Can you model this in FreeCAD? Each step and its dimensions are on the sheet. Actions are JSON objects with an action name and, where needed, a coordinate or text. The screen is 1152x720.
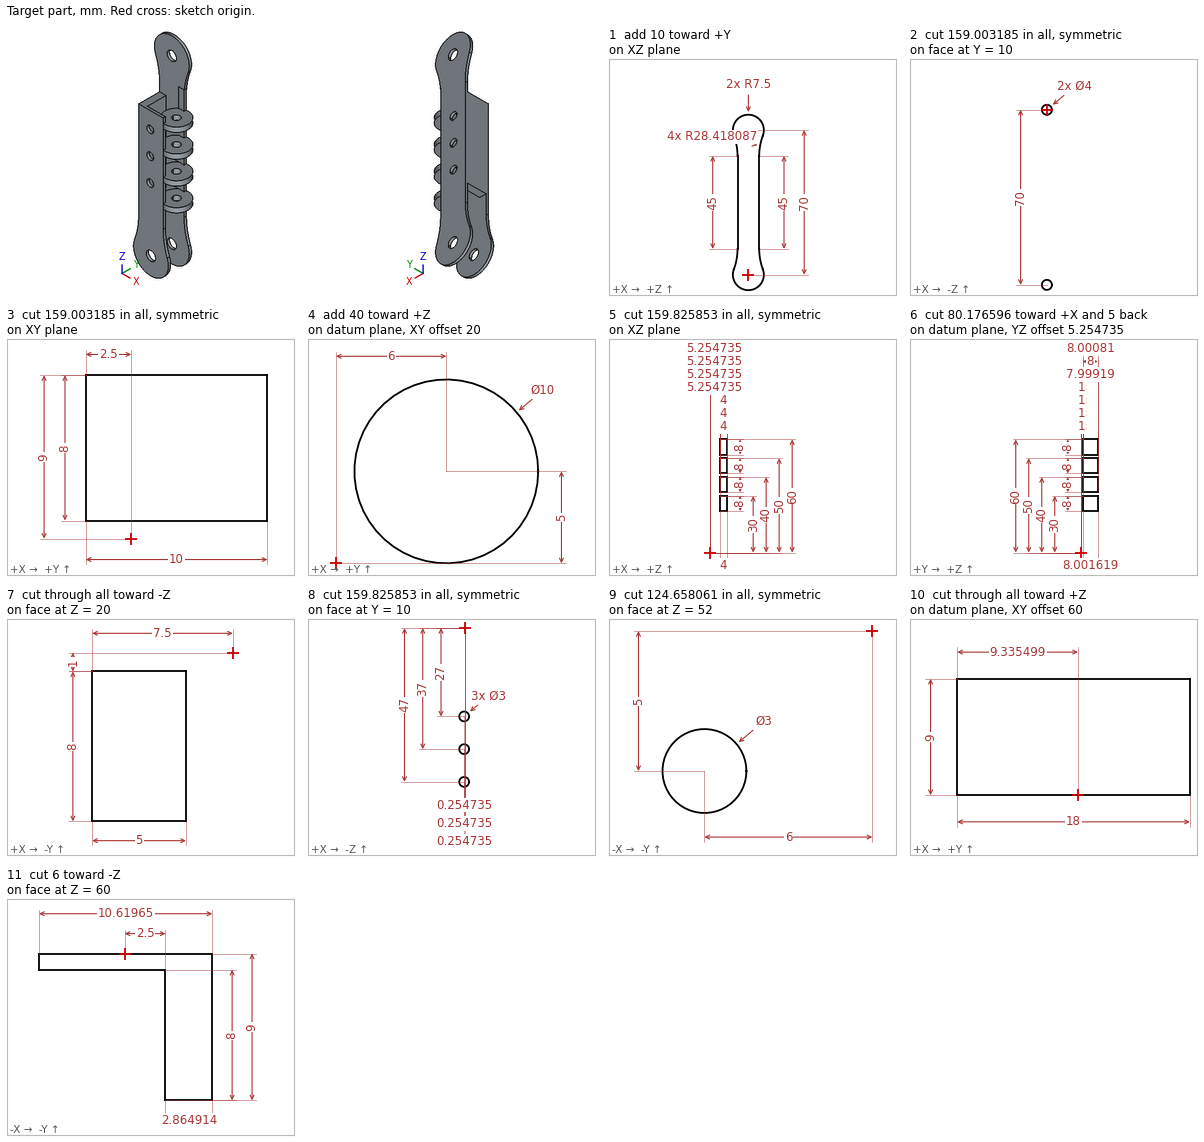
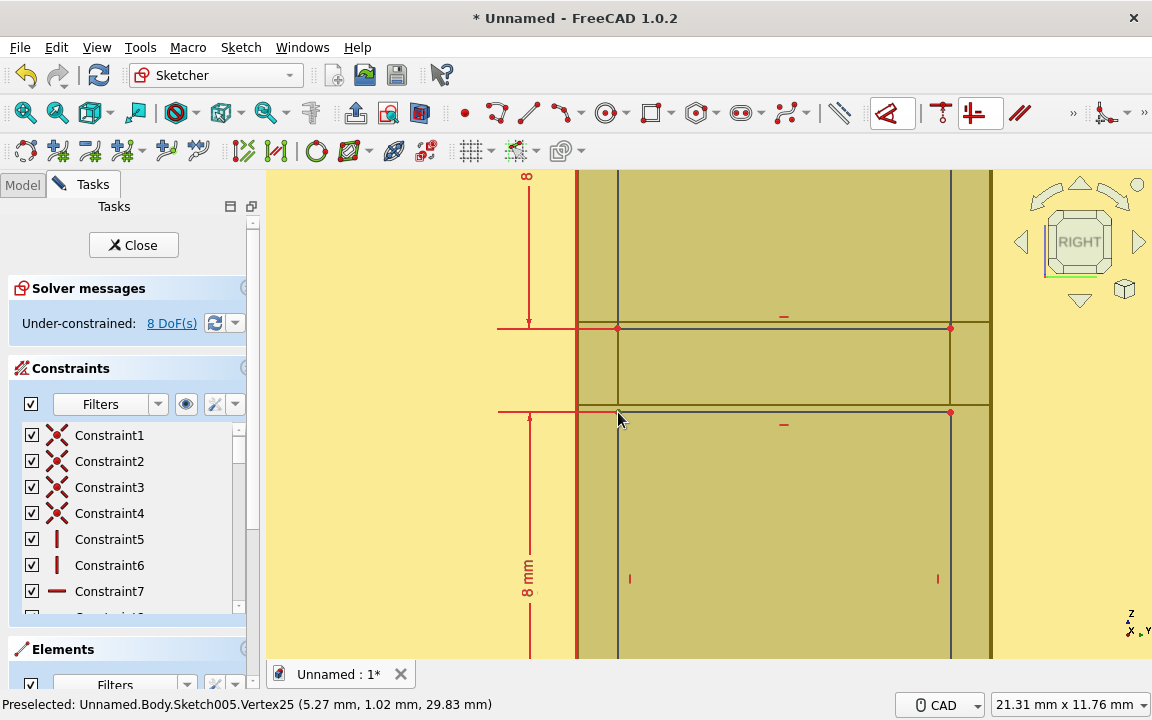
{"action": "left_click", "coordinate": [910, 114]}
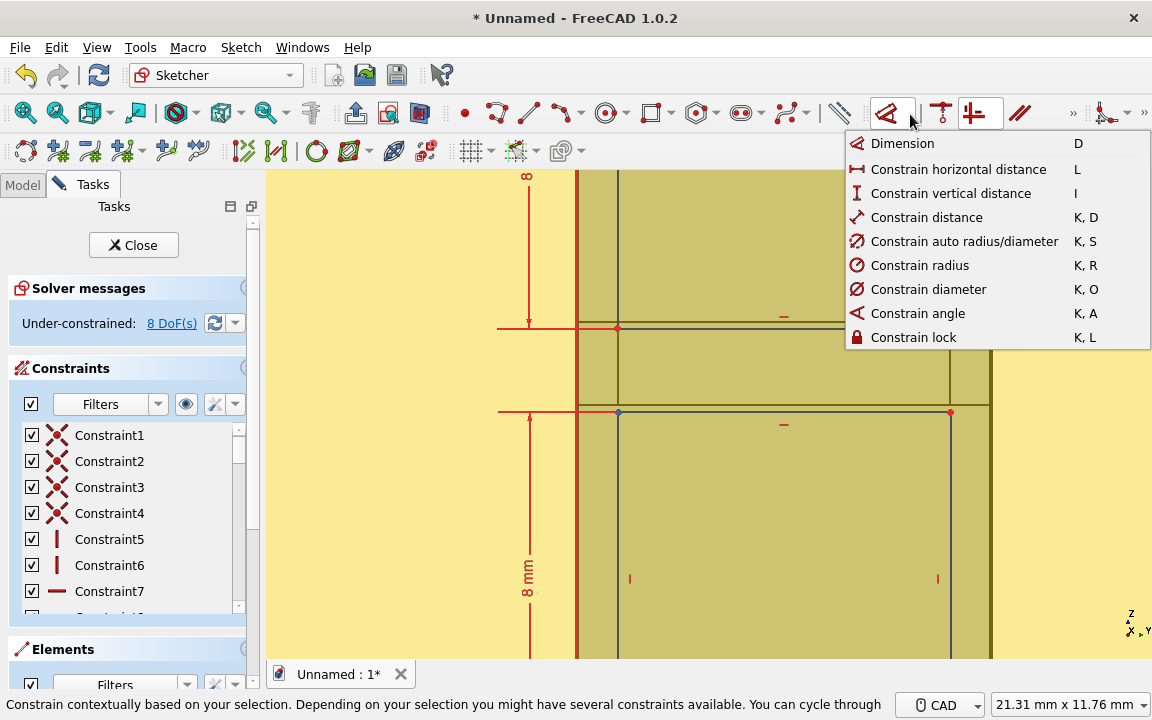
{"action": "left_click", "coordinate": [998, 169]}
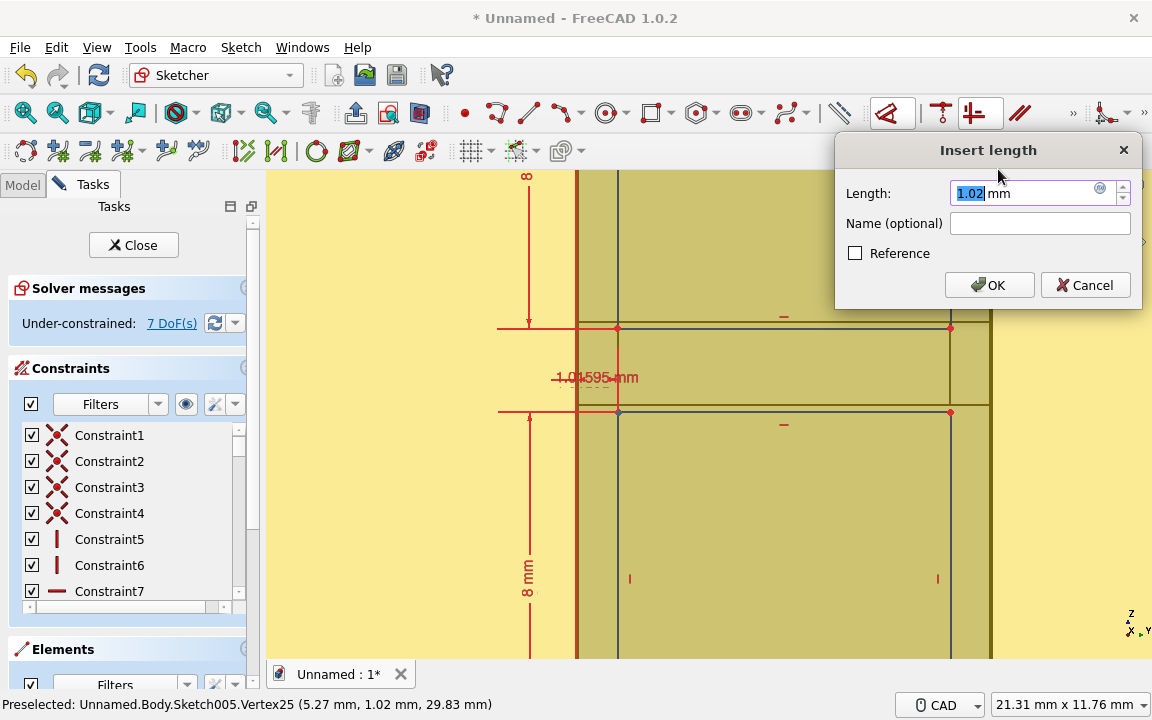
{"action": "type", "text": "1"}
{"action": "key", "text": "Return"}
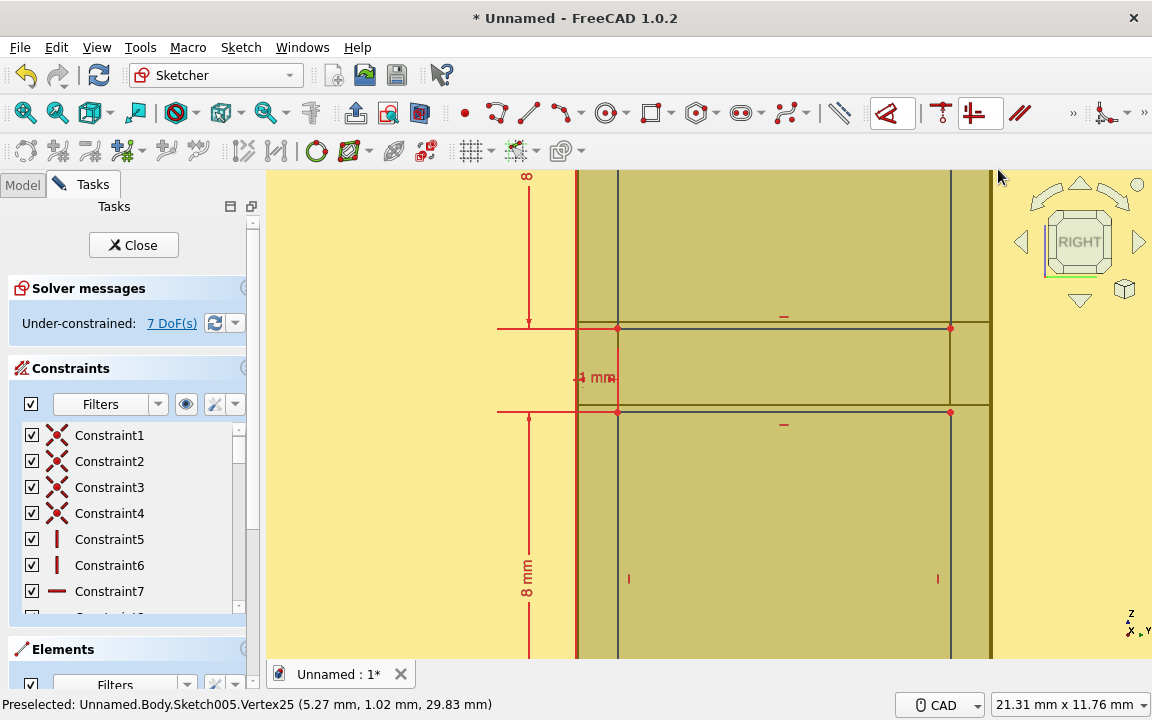
{"action": "scroll", "coordinate": [621, 416], "scroll_direction": "down", "scroll_amount": 10}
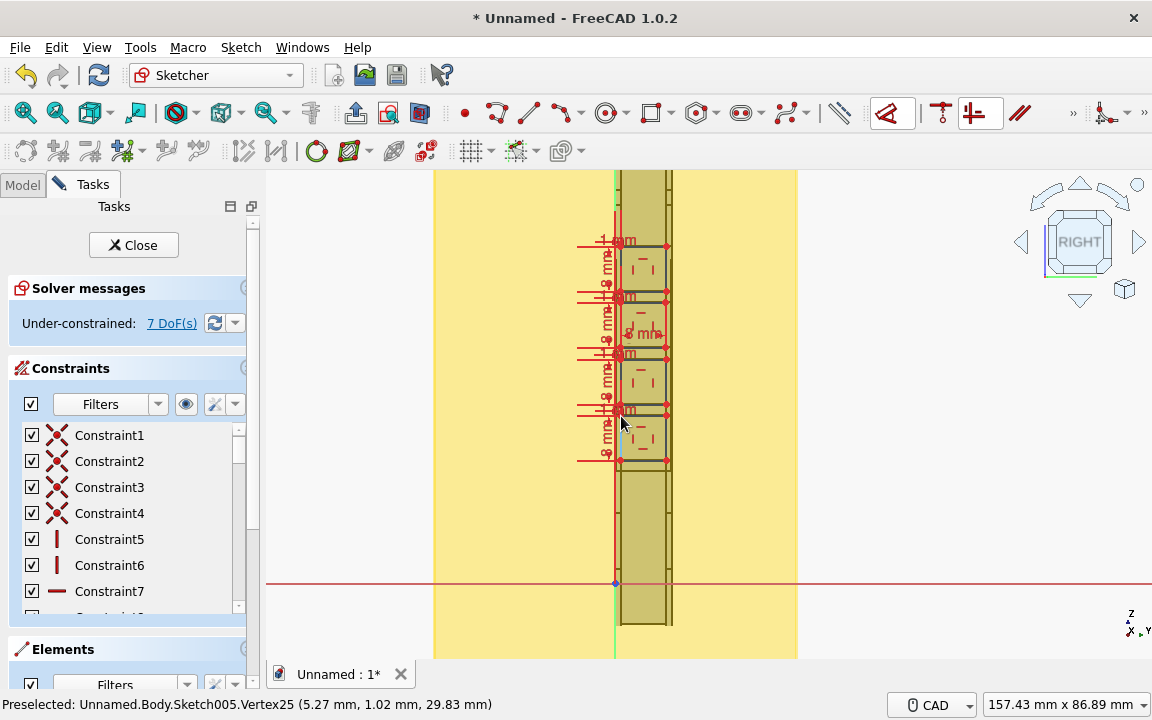
{"action": "left_click", "coordinate": [621, 247]}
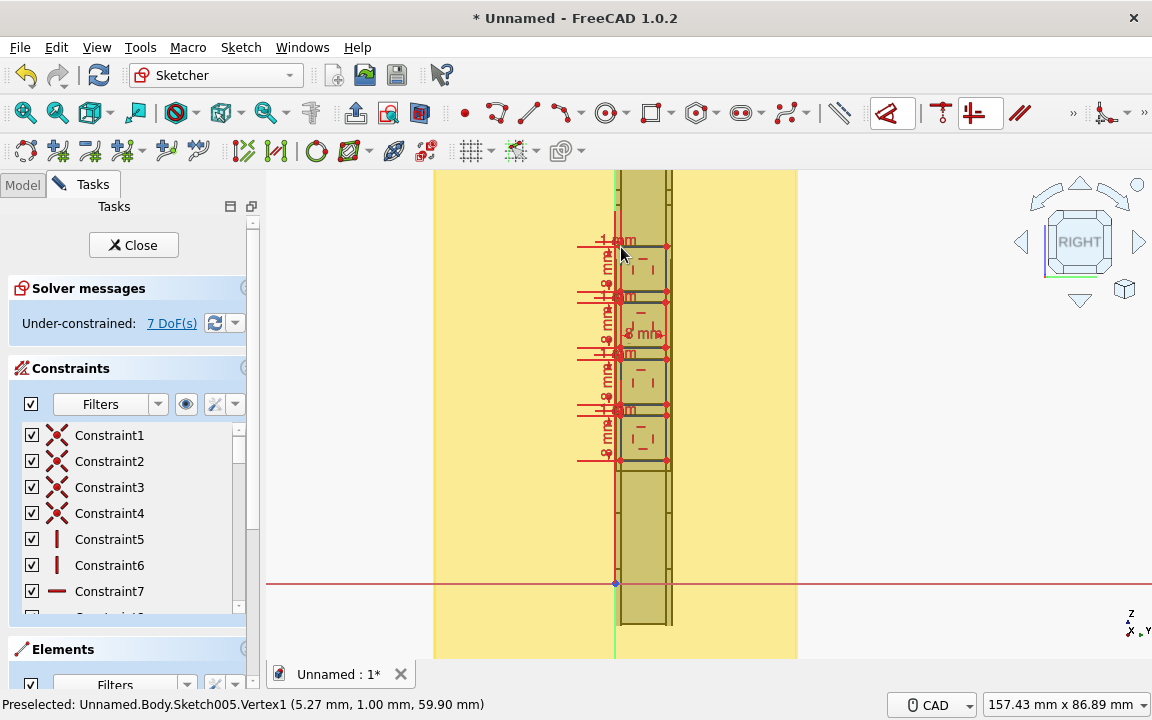
{"action": "left_click", "coordinate": [910, 114]}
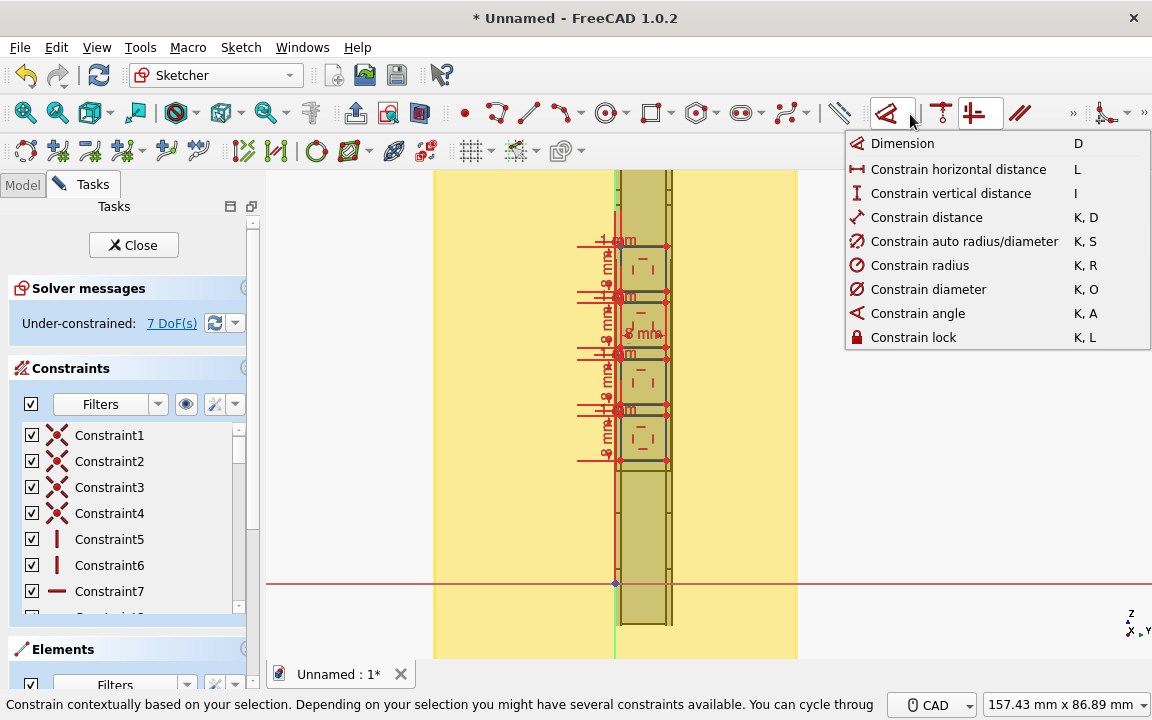
{"action": "left_click", "coordinate": [998, 193]}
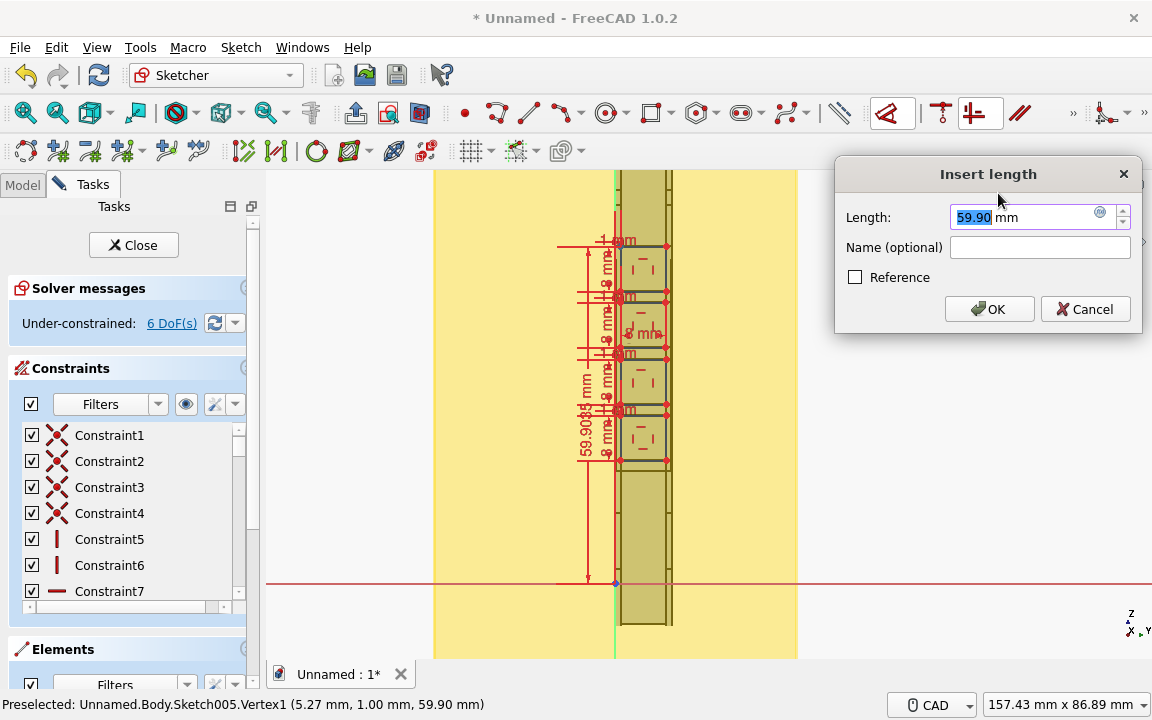
{"action": "type", "text": "60"}
{"action": "key", "text": "Return"}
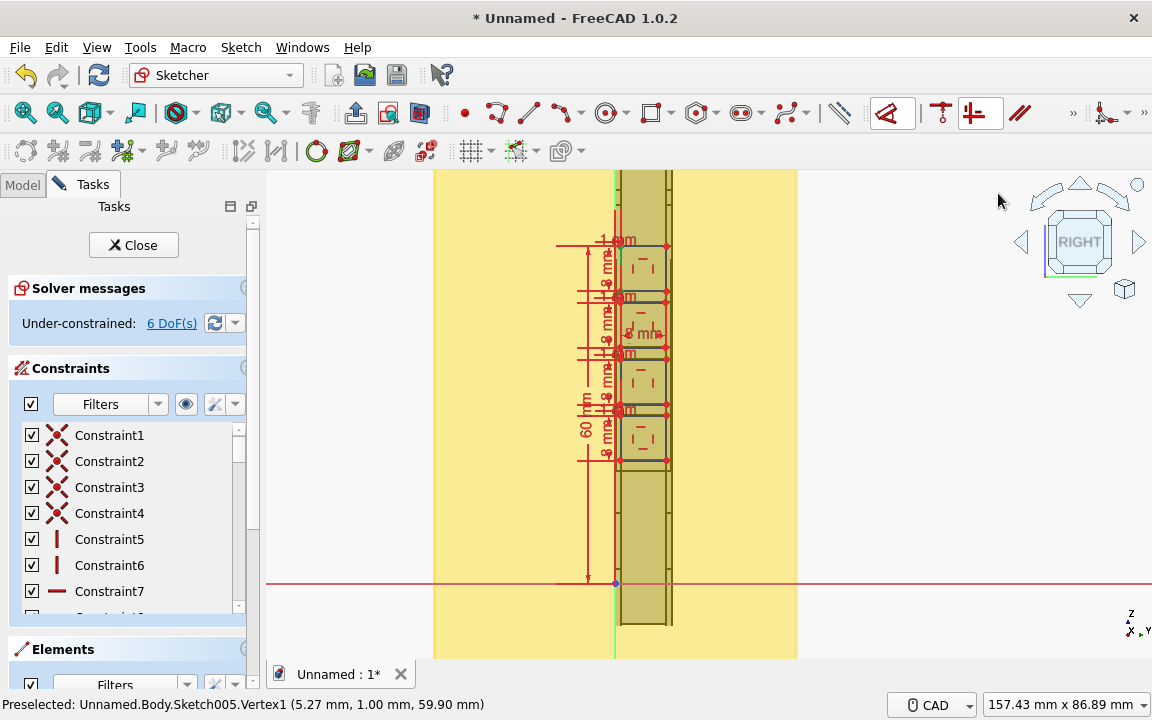
{"action": "left_click", "coordinate": [621, 303]}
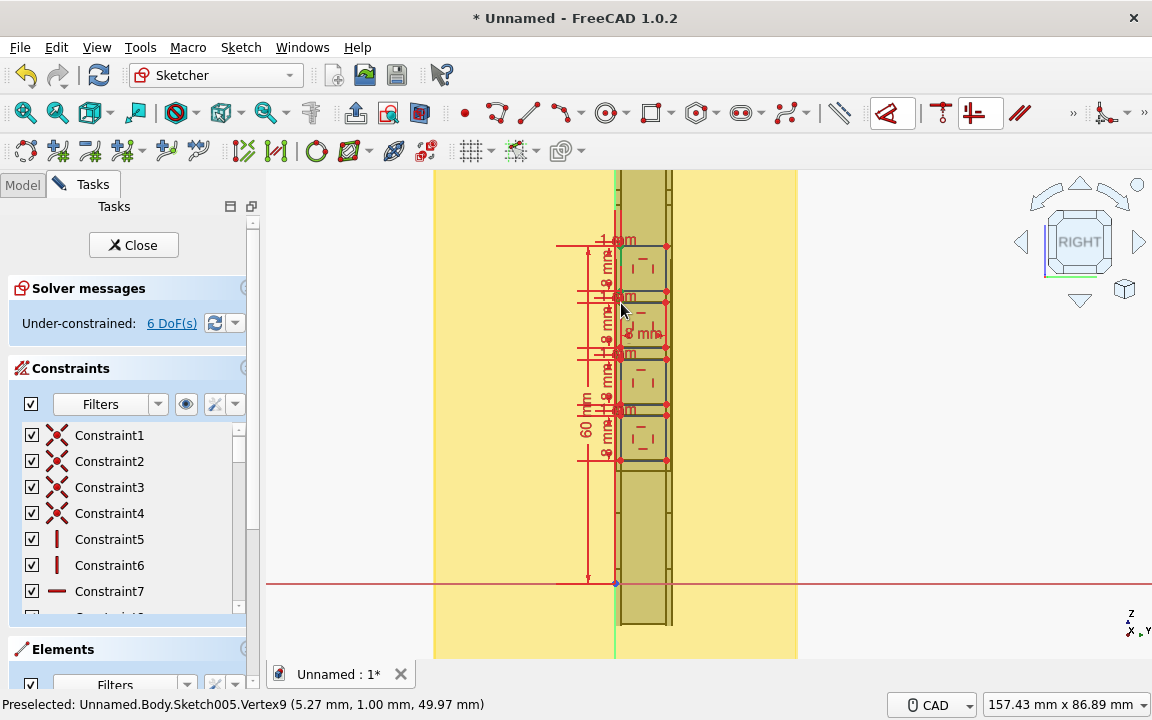
{"action": "key", "text": "i"}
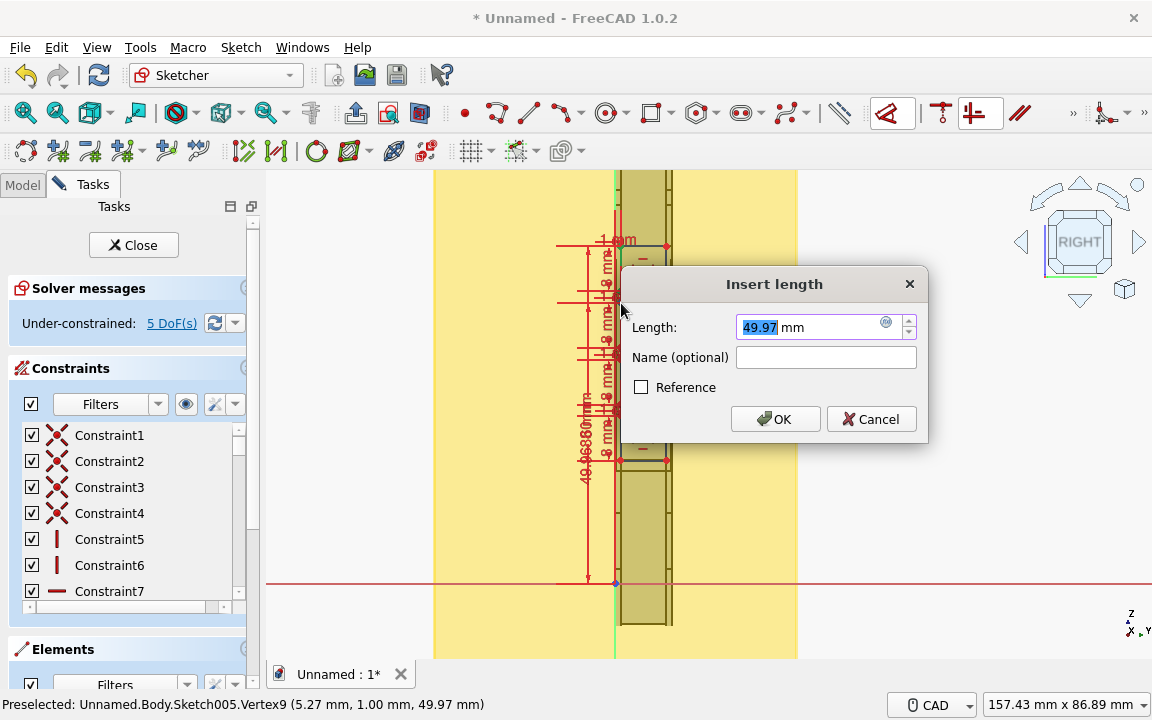
{"action": "type", "text": "50"}
{"action": "key", "text": "Return"}